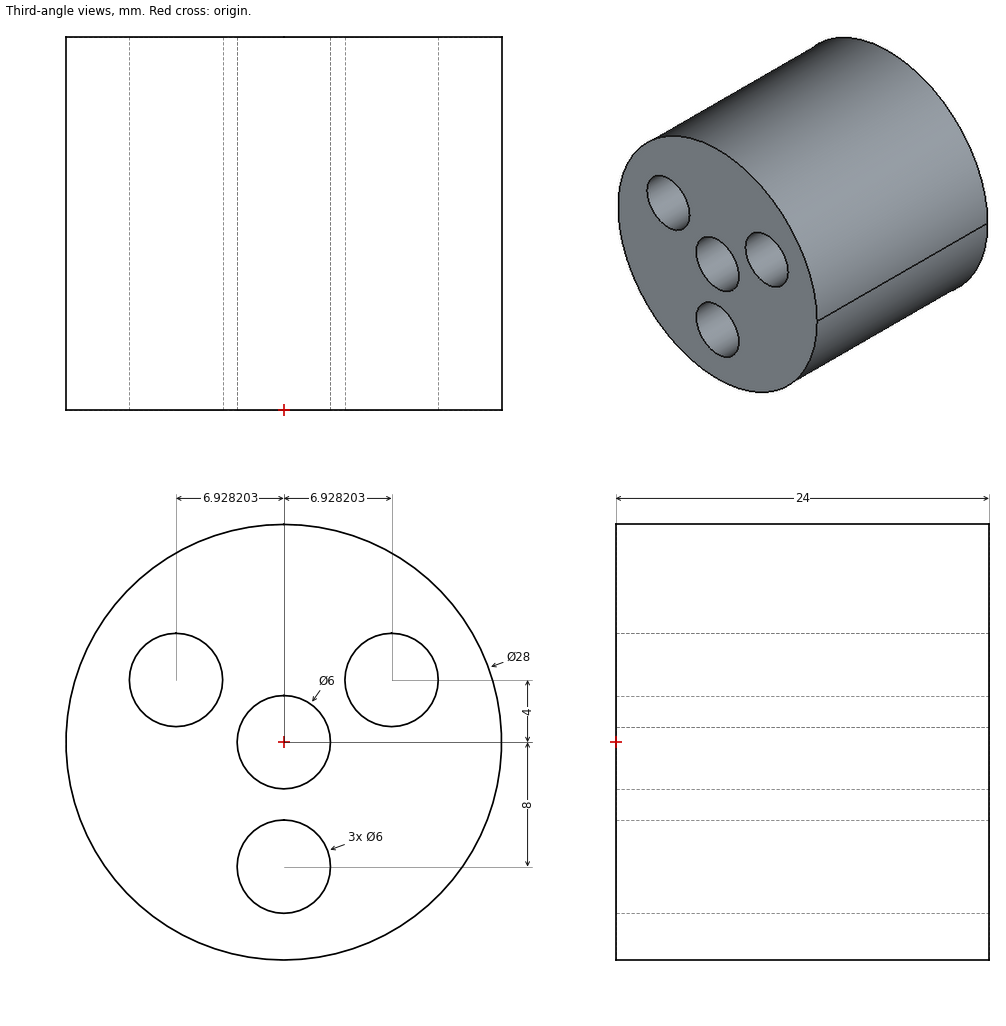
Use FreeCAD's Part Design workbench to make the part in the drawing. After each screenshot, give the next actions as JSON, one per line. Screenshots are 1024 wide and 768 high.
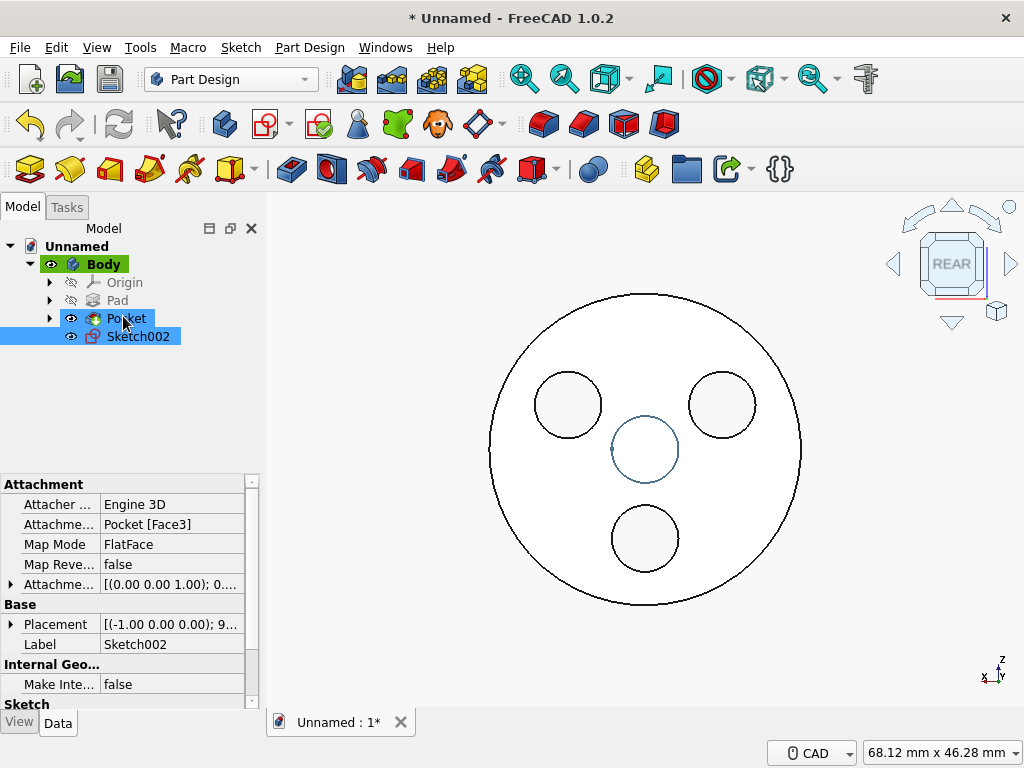
{"action": "left_click", "coordinate": [292, 170]}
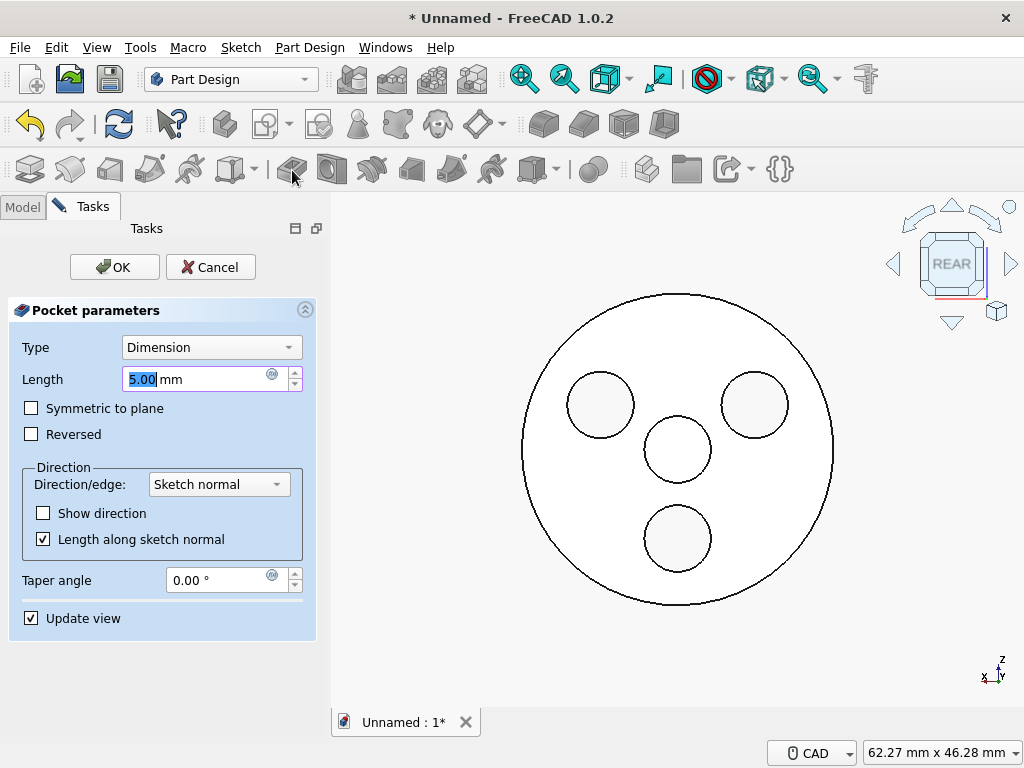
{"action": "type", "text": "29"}
{"action": "key", "text": "Tab"}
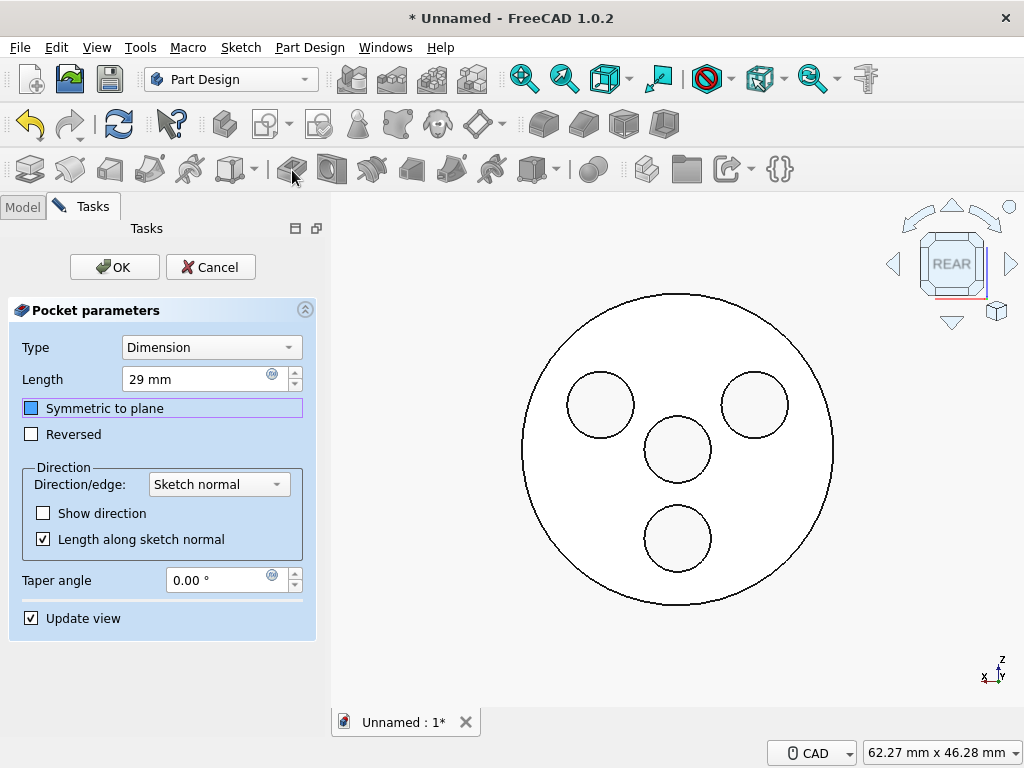
{"action": "left_click", "coordinate": [115, 267]}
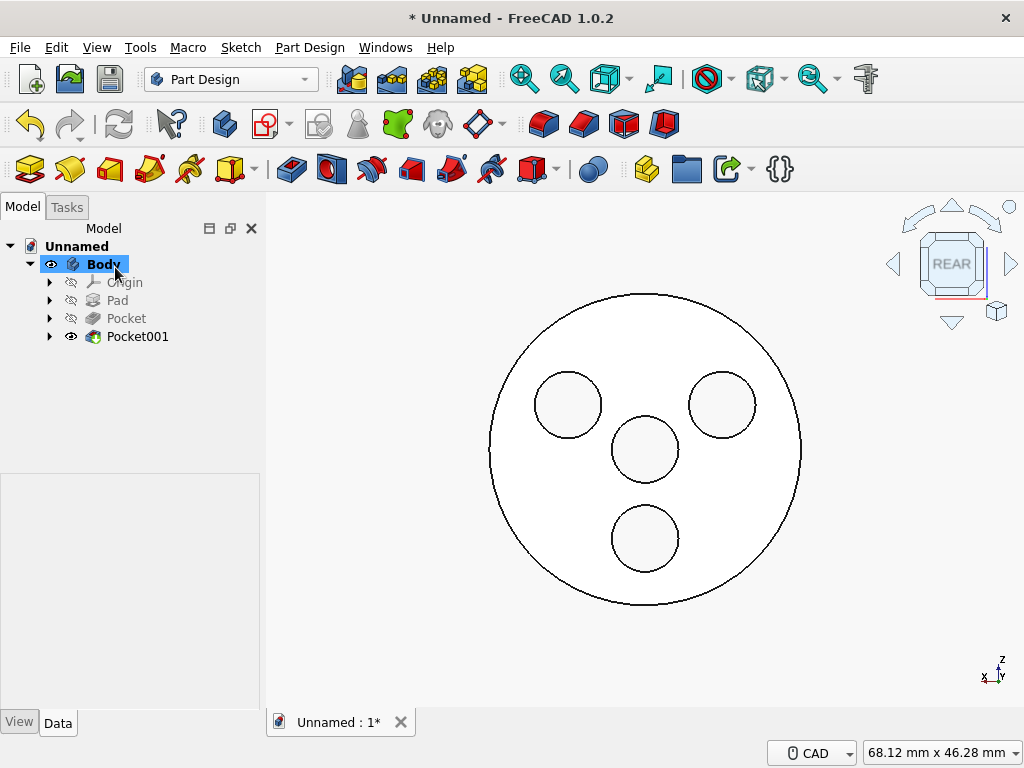
{"action": "key", "text": "0"}